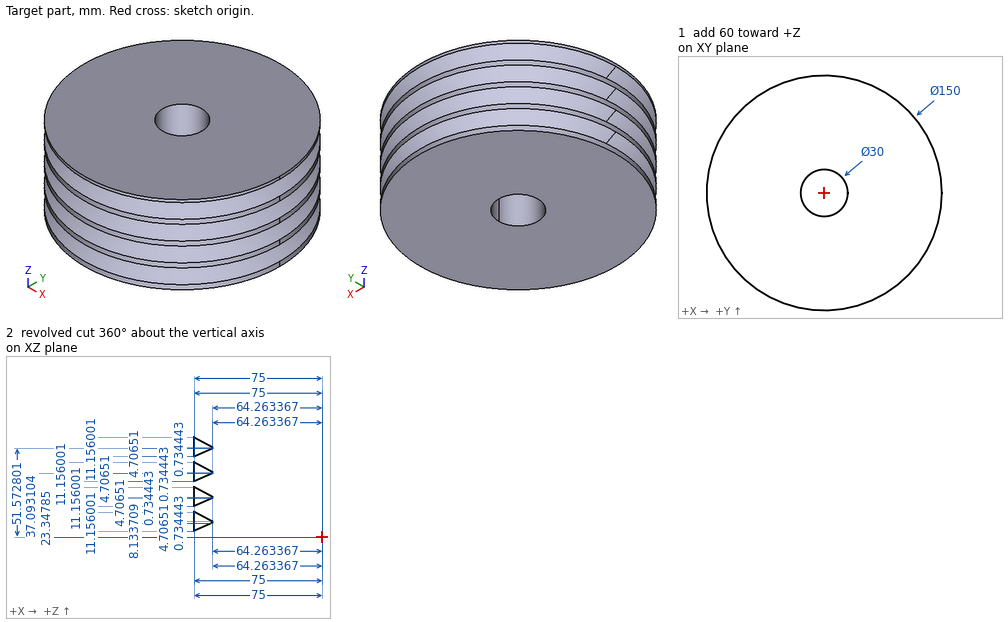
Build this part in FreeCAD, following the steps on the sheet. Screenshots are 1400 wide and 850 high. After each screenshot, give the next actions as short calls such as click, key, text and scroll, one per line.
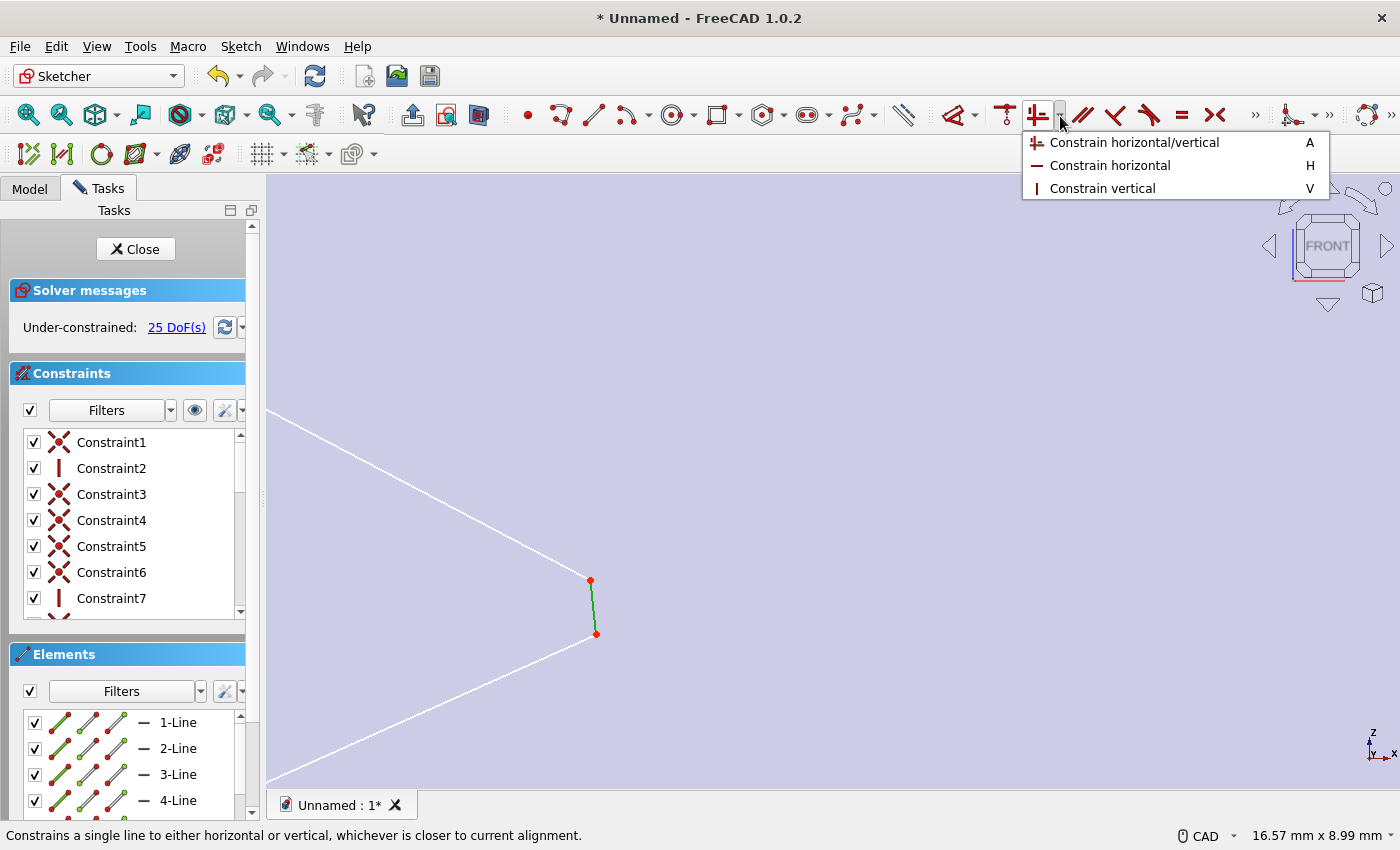
click(1176, 188)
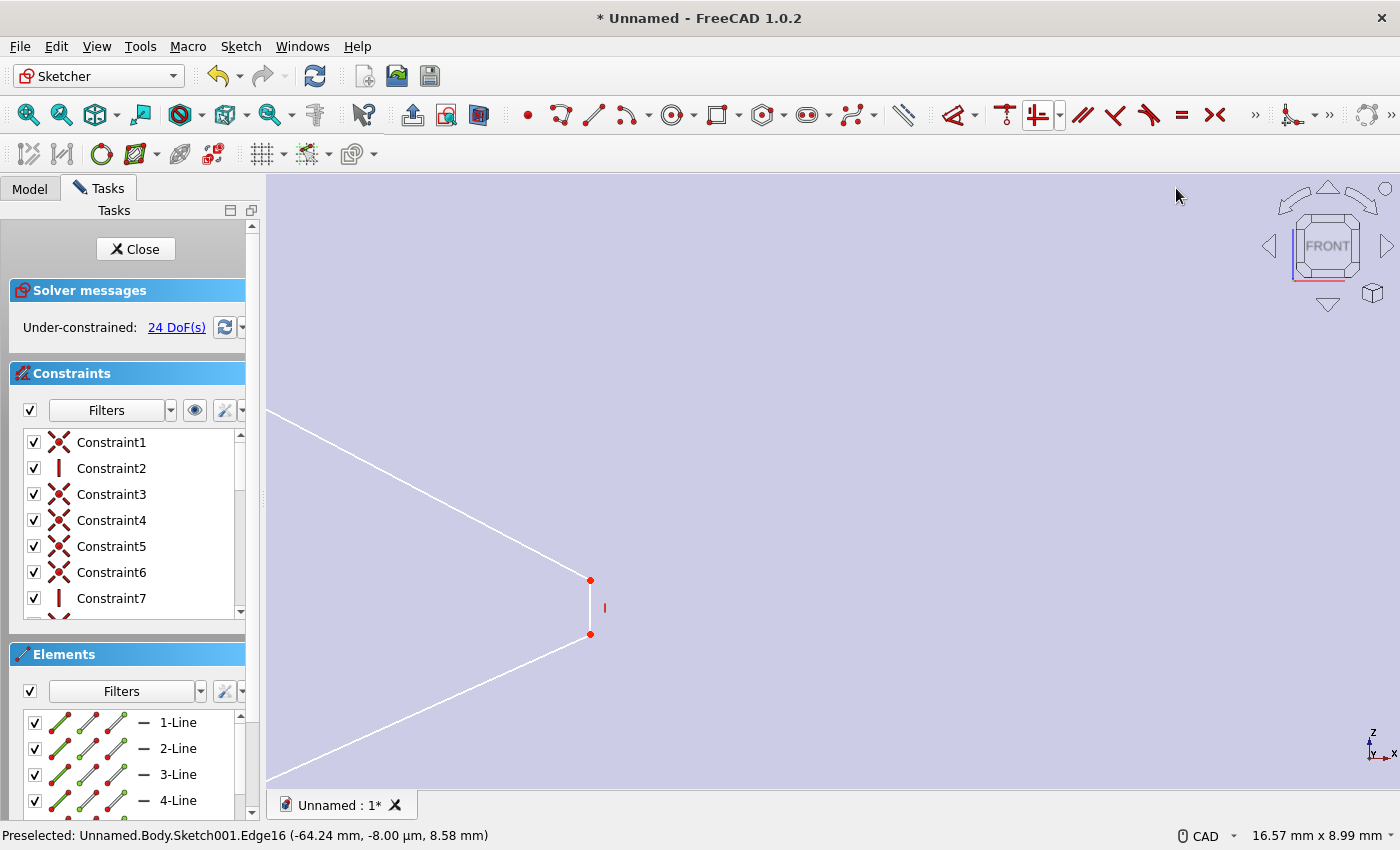
click(952, 116)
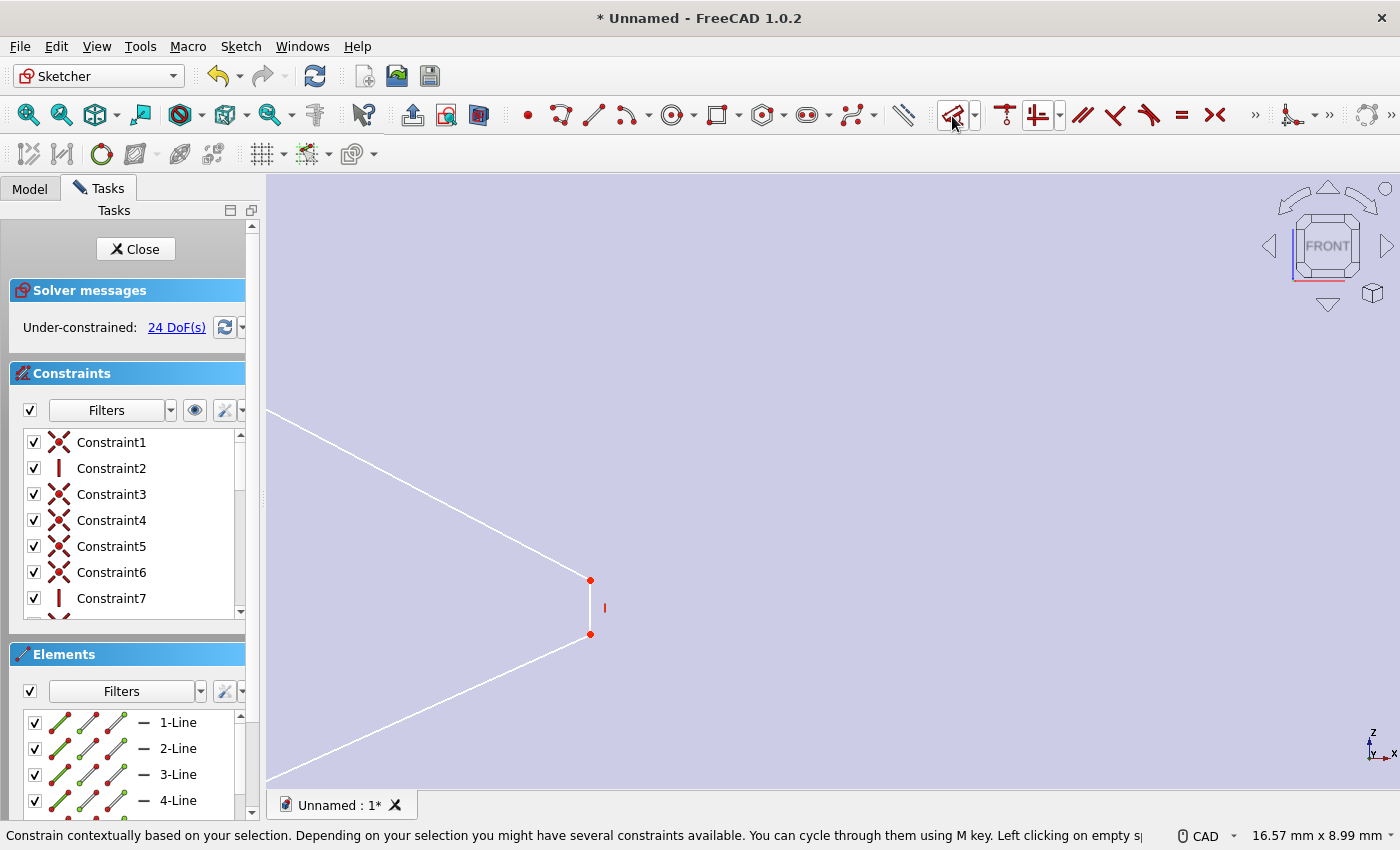
scroll(599, 609, down, 12)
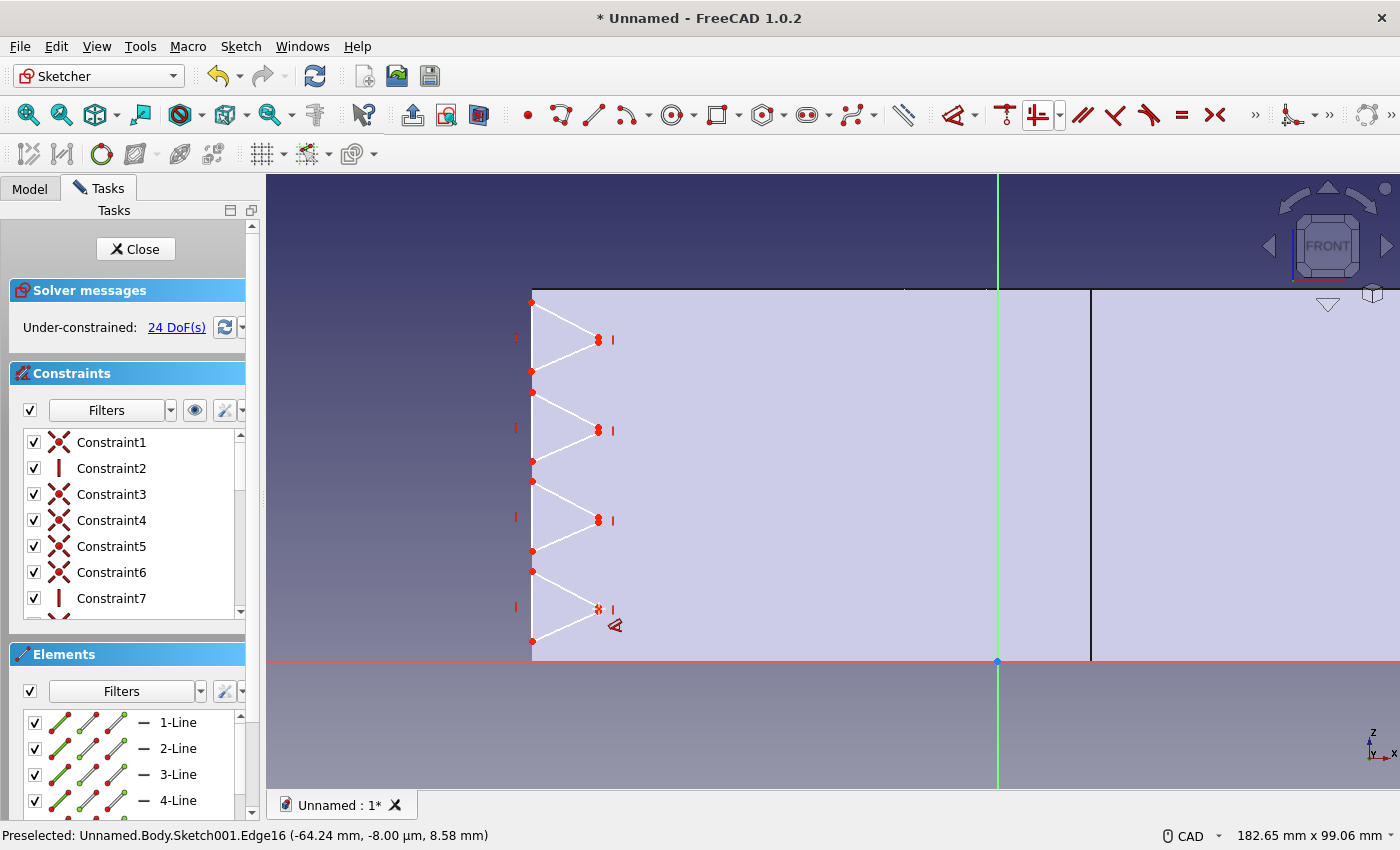
click(532, 372)
click(765, 696)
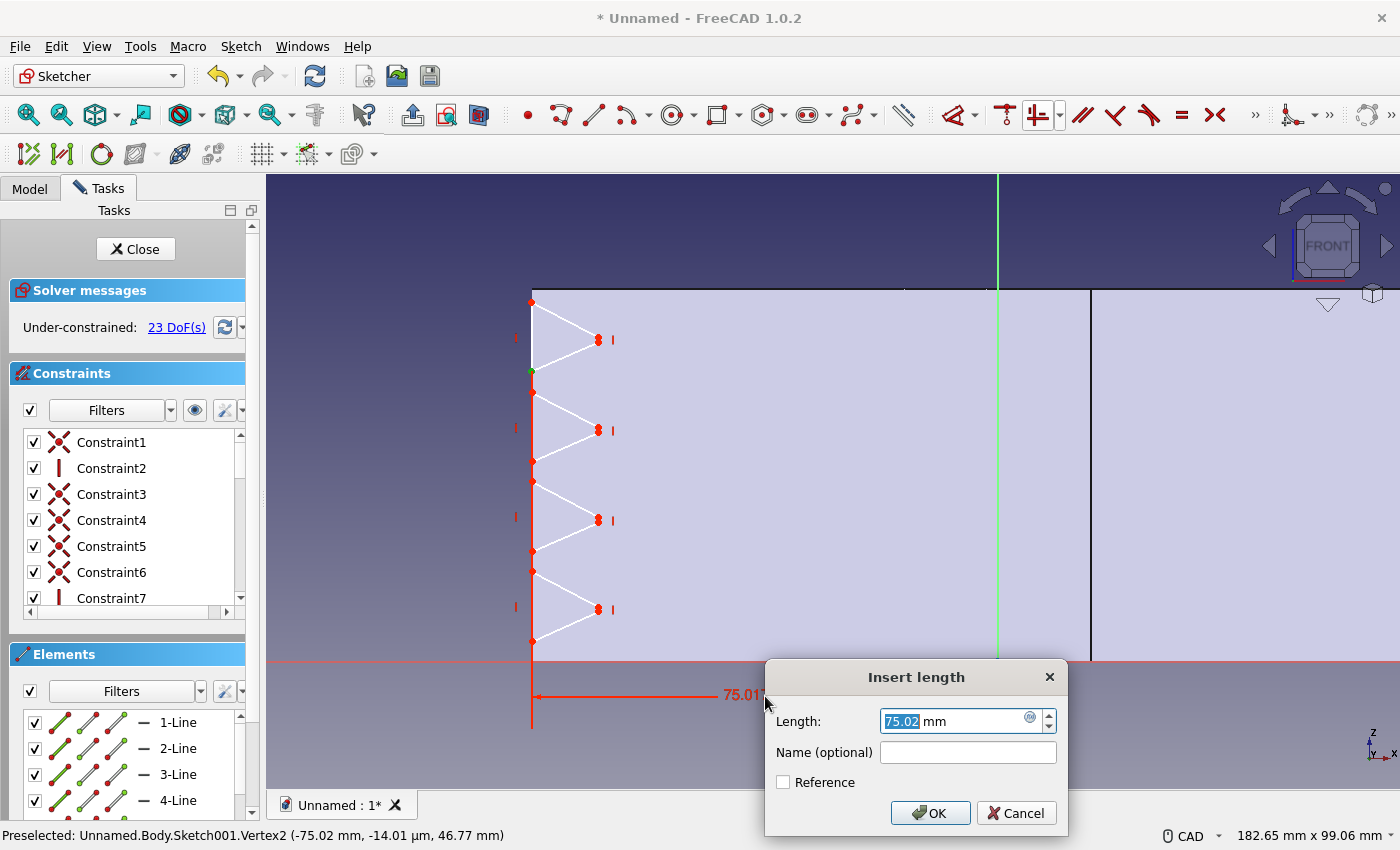
text(75)
key(Return)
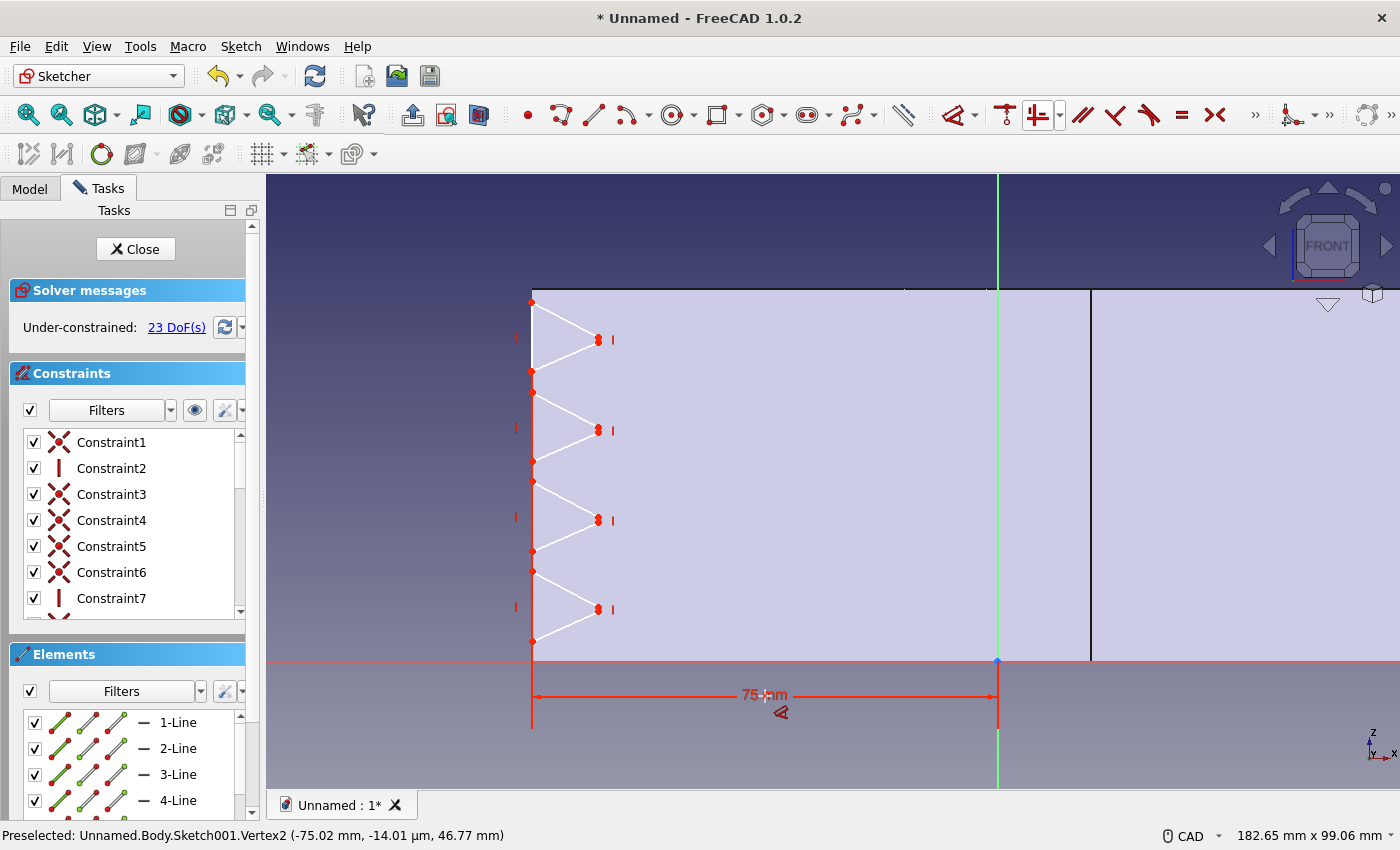
click(532, 462)
click(658, 696)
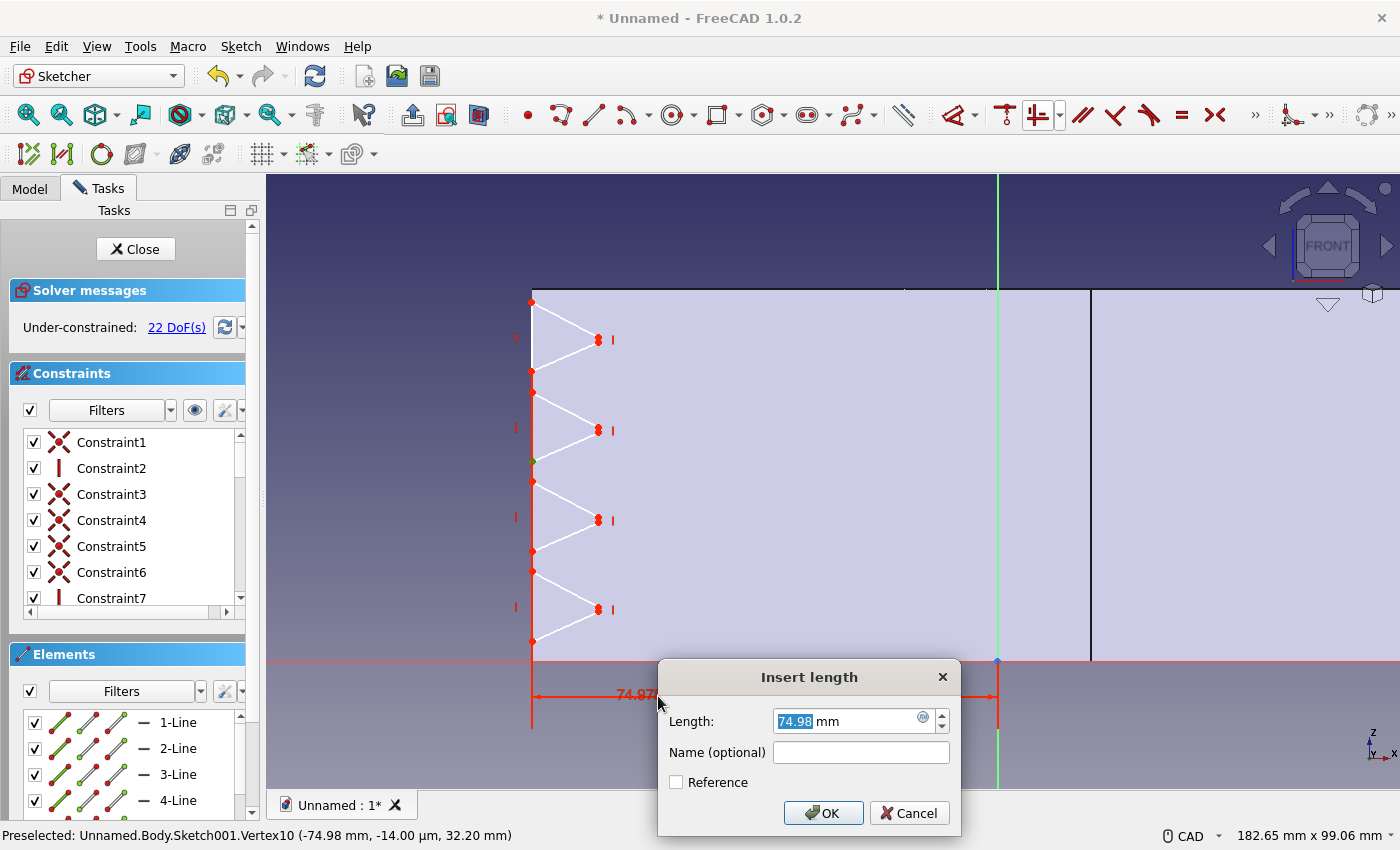
text(75)
key(Return)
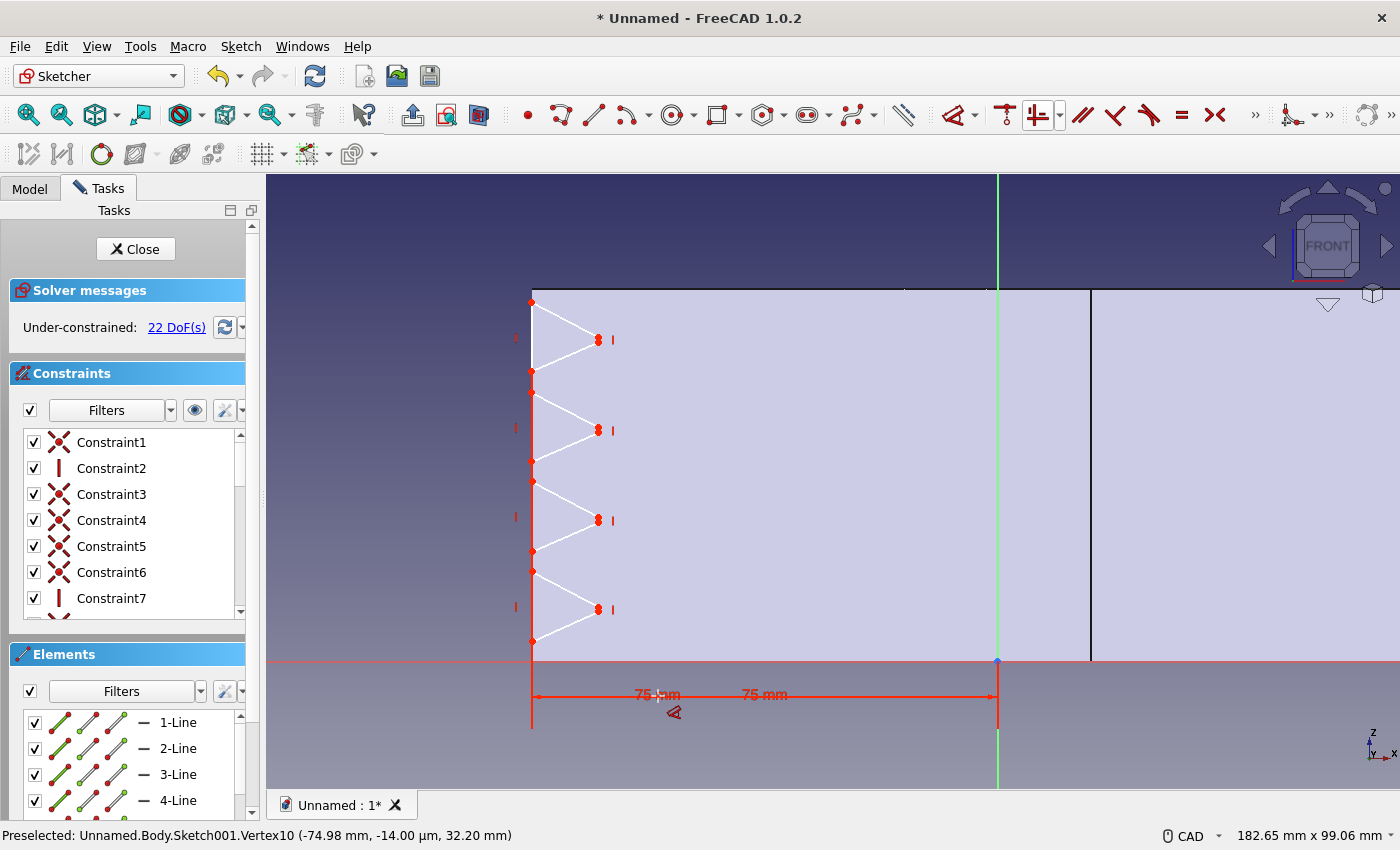
click(532, 552)
click(872, 696)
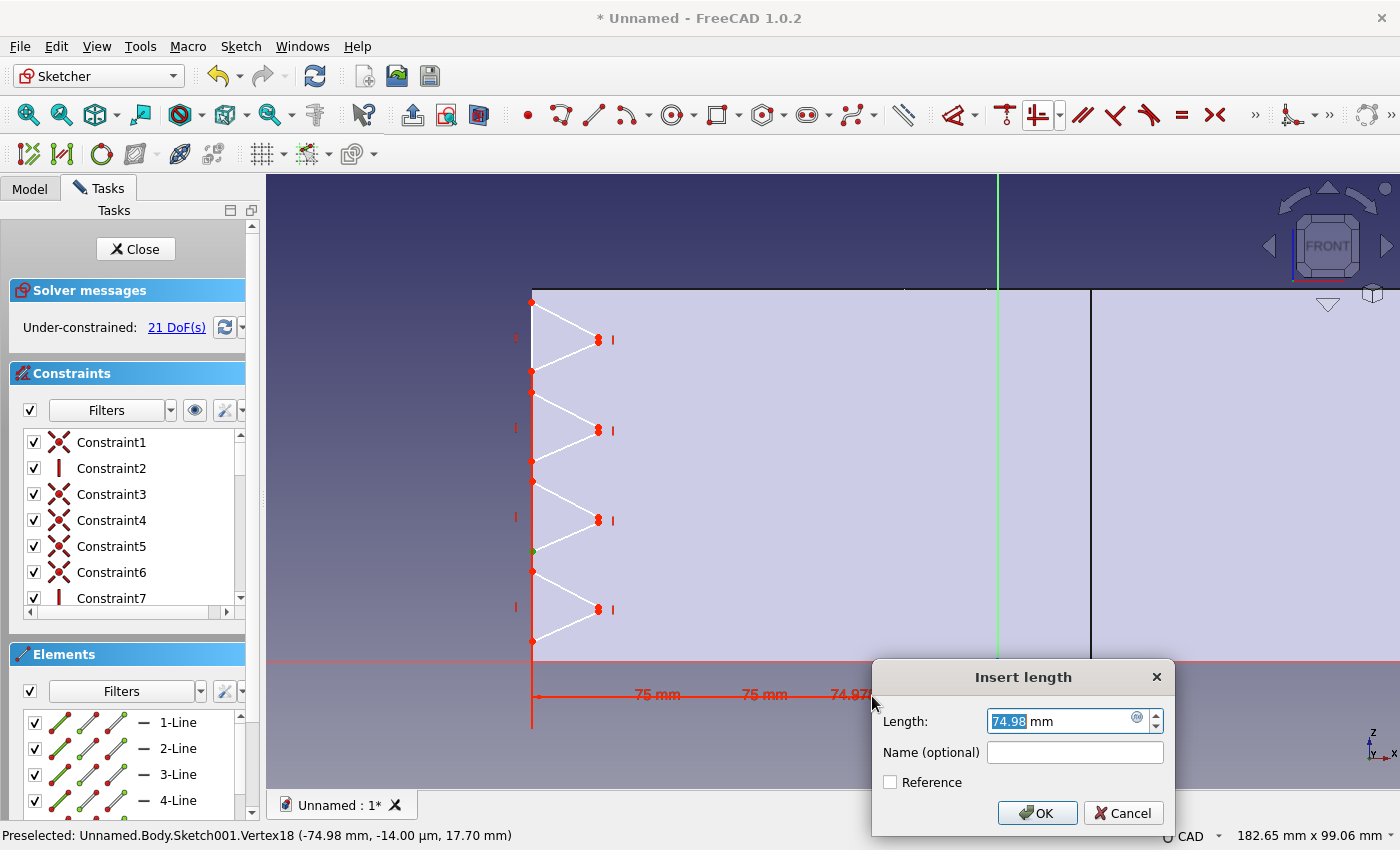
text(75)
key(Return)